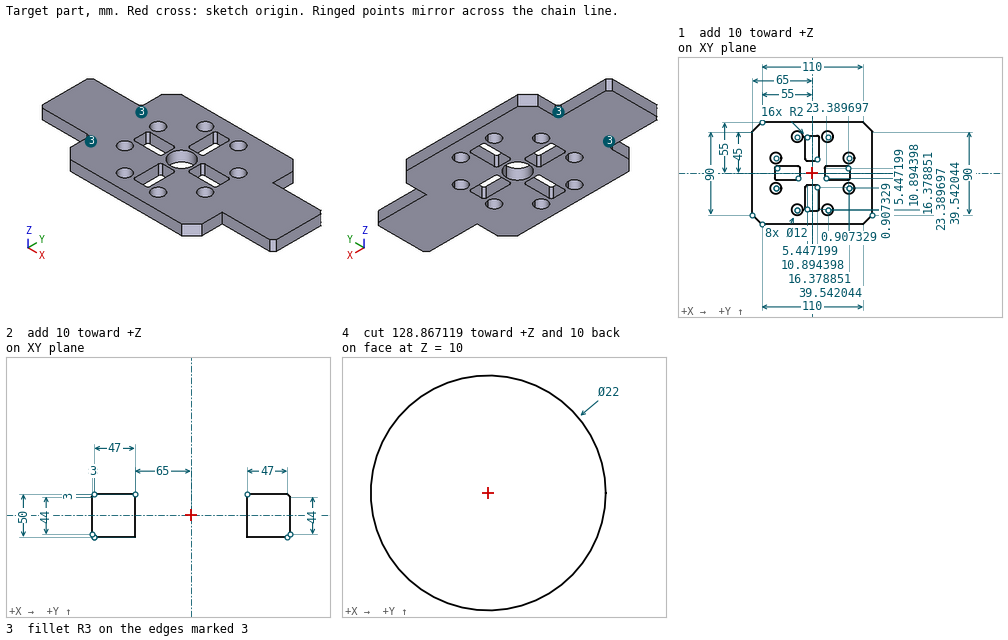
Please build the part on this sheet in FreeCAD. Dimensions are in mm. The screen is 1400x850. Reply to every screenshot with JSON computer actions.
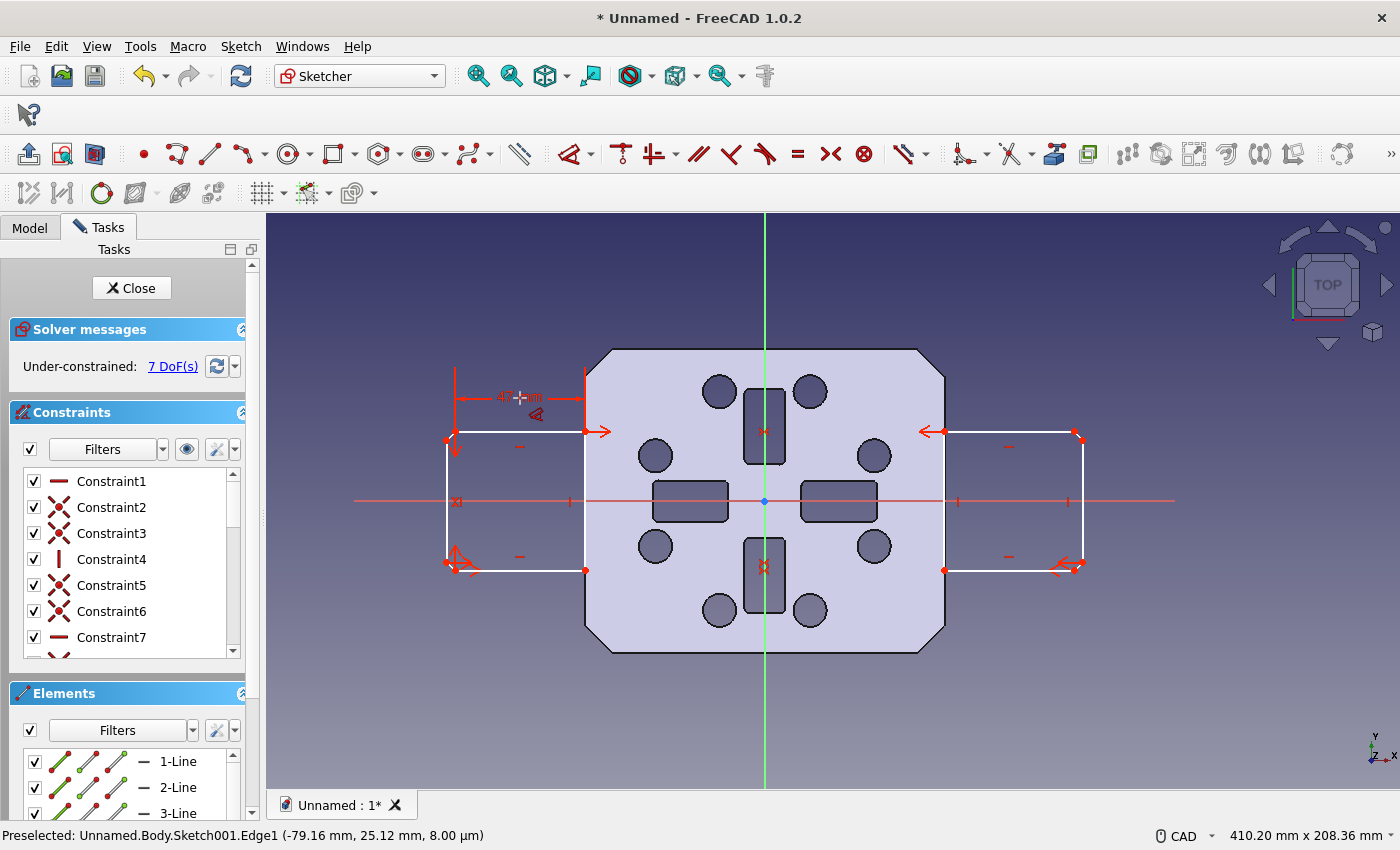
{"action": "left_click", "coordinate": [447, 477]}
{"action": "left_click", "coordinate": [413, 474]}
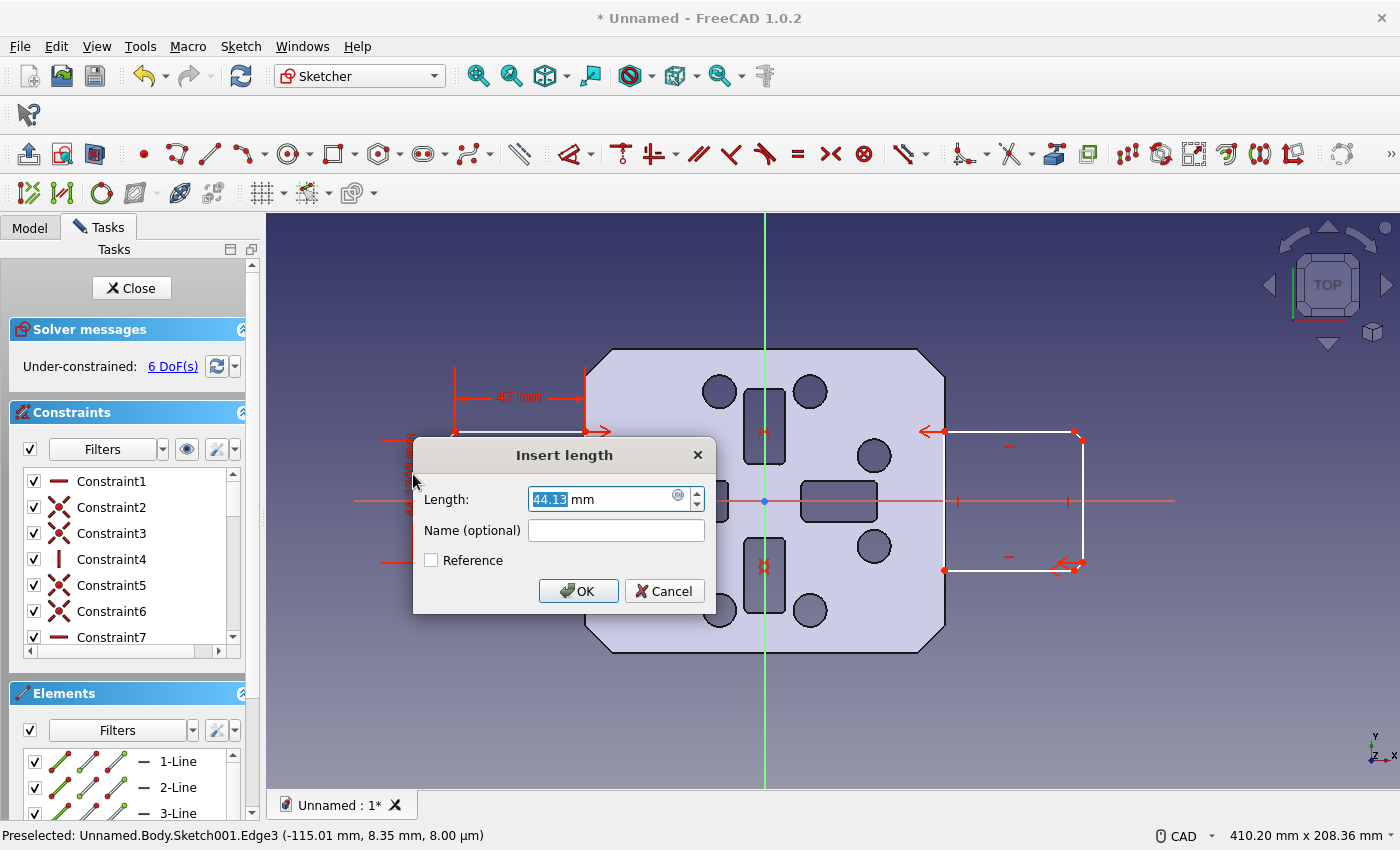
{"action": "type", "text": "44"}
{"action": "key", "text": "Return"}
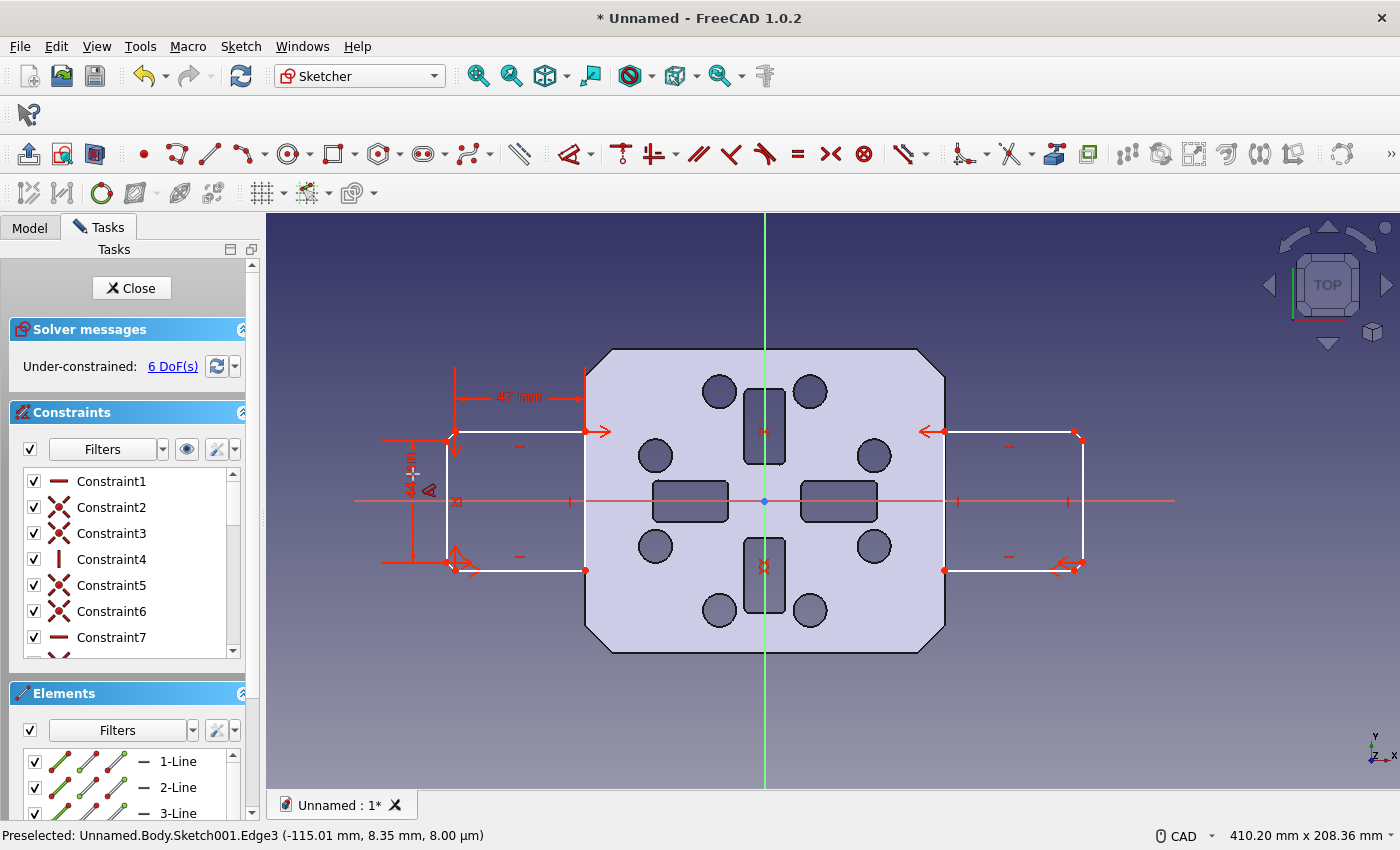
{"action": "left_click", "coordinate": [585, 529]}
{"action": "left_click", "coordinate": [551, 469]}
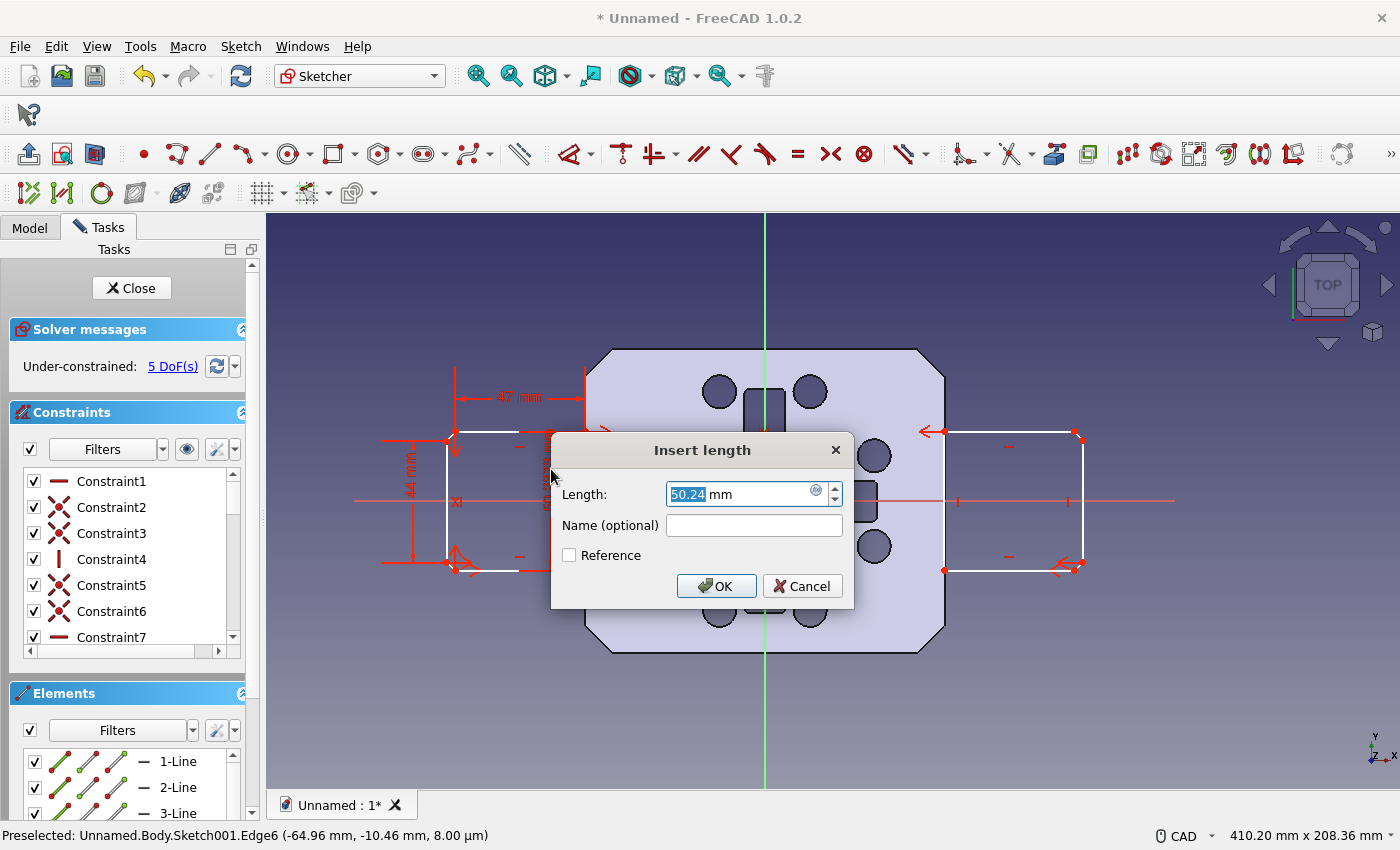
{"action": "type", "text": "50"}
{"action": "key", "text": "Return"}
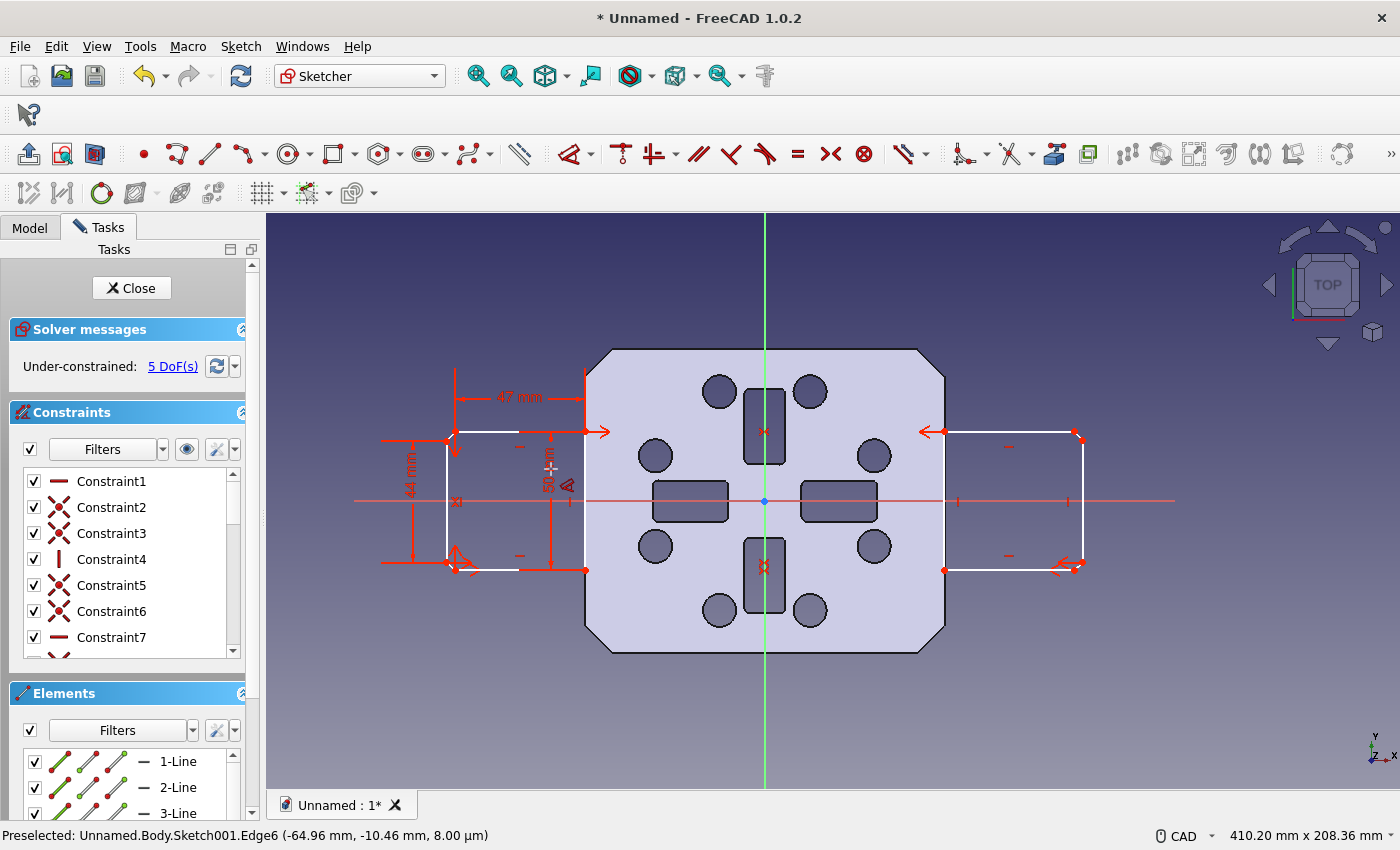
{"action": "left_click", "coordinate": [1083, 526]}
{"action": "left_click", "coordinate": [1117, 474]}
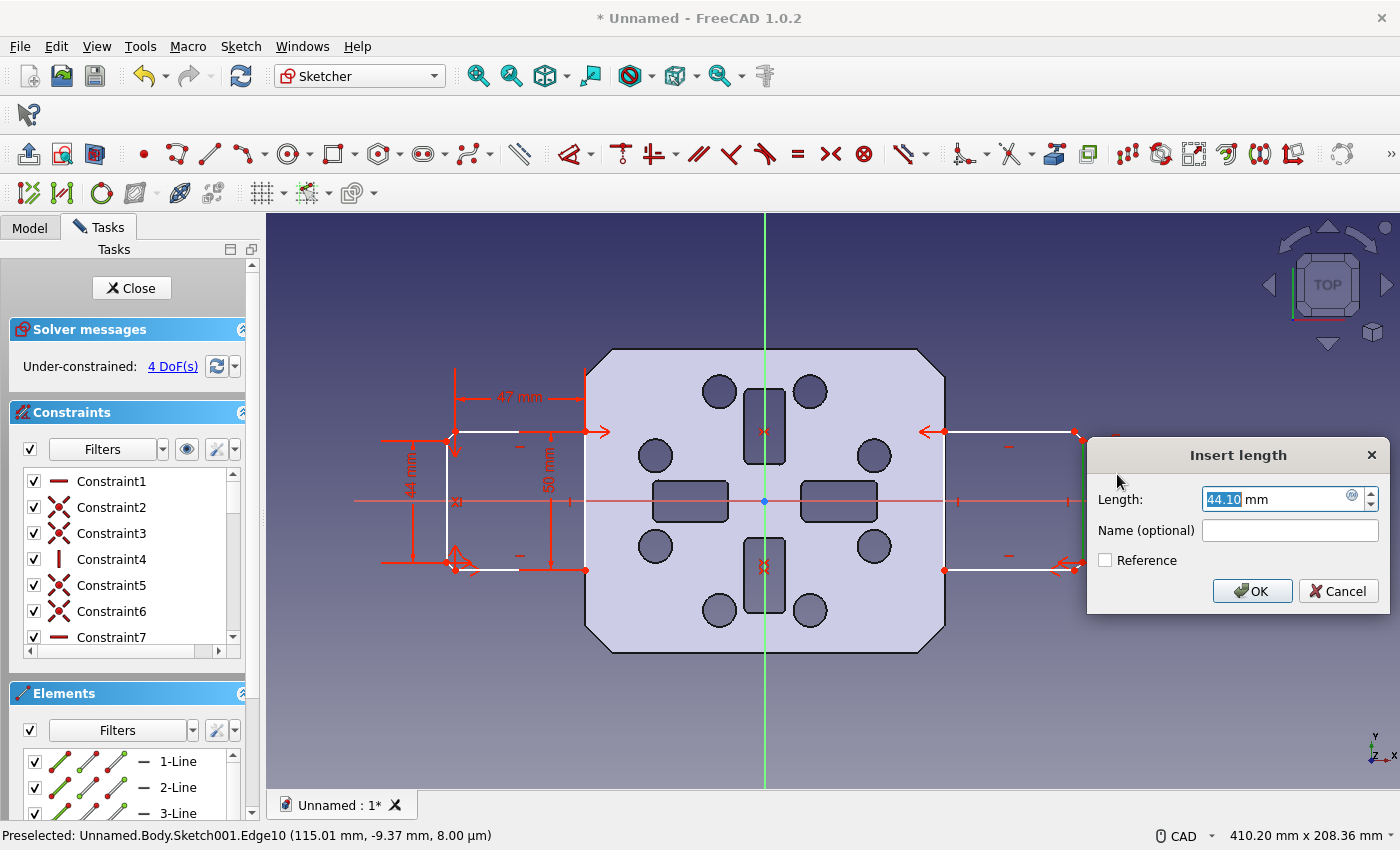
{"action": "type", "text": "44"}
{"action": "key", "text": "Return"}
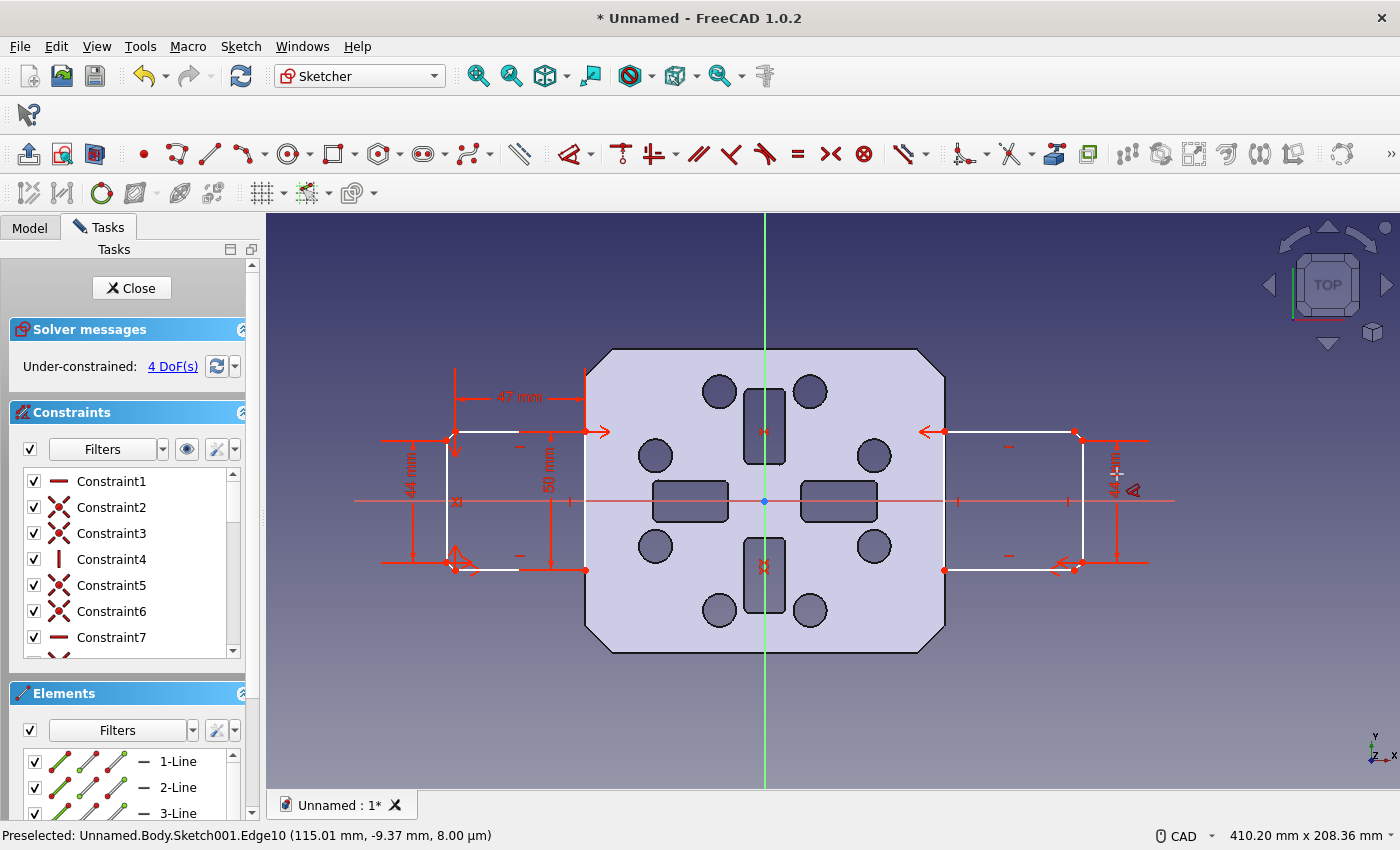
{"action": "left_click", "coordinate": [1035, 432]}
{"action": "left_click", "coordinate": [1009, 398]}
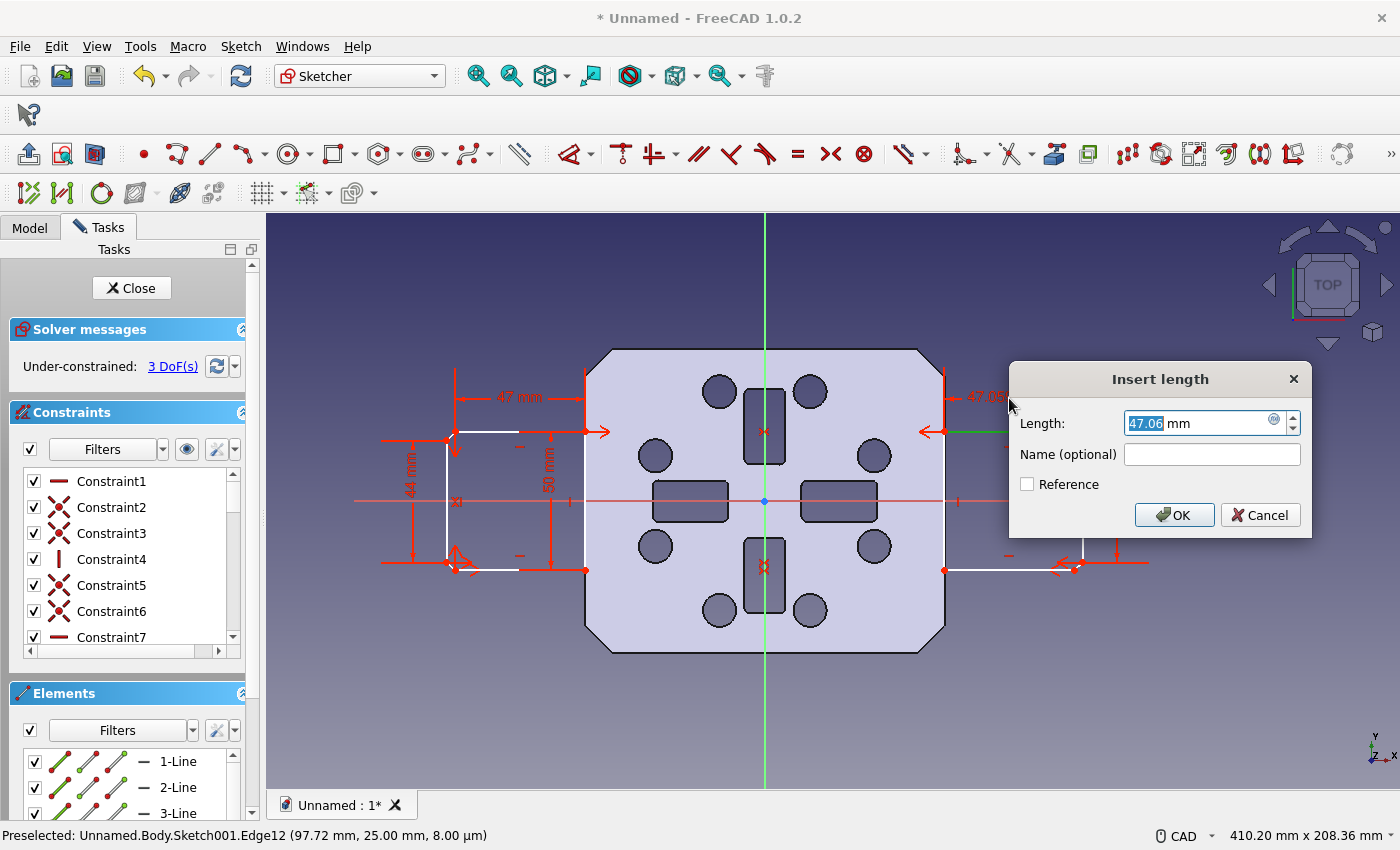
{"action": "type", "text": "47"}
{"action": "key", "text": "Return"}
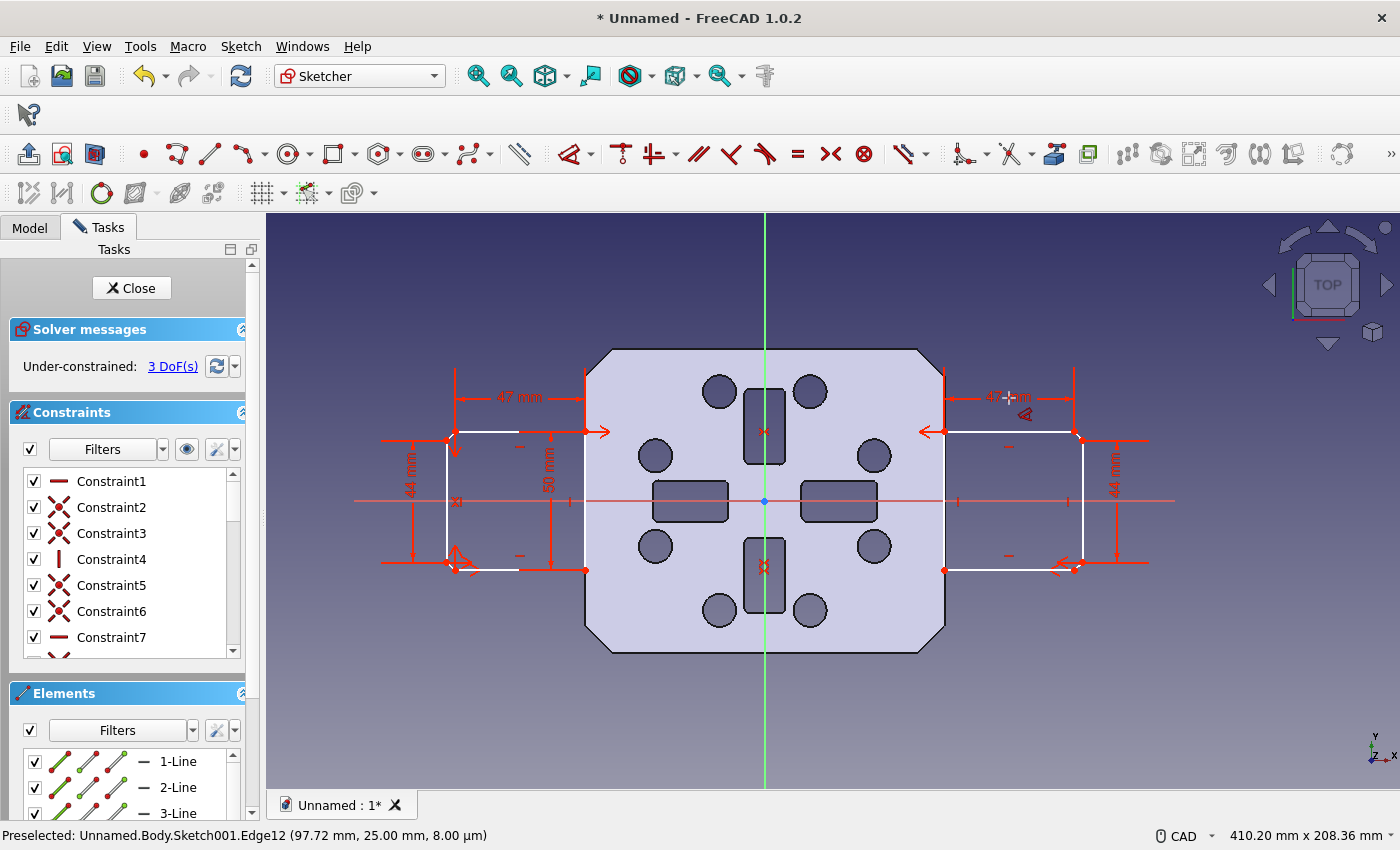
{"action": "scroll", "coordinate": [451, 436], "scroll_direction": "up", "scroll_amount": 8}